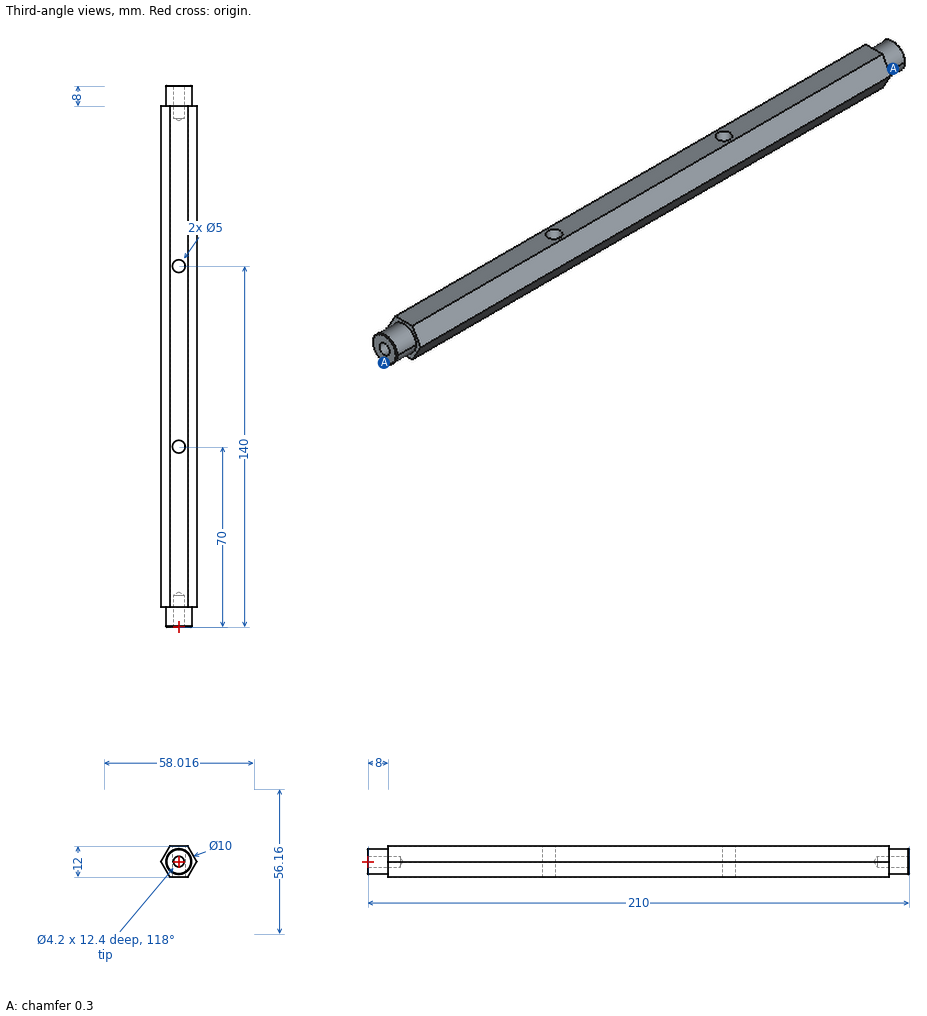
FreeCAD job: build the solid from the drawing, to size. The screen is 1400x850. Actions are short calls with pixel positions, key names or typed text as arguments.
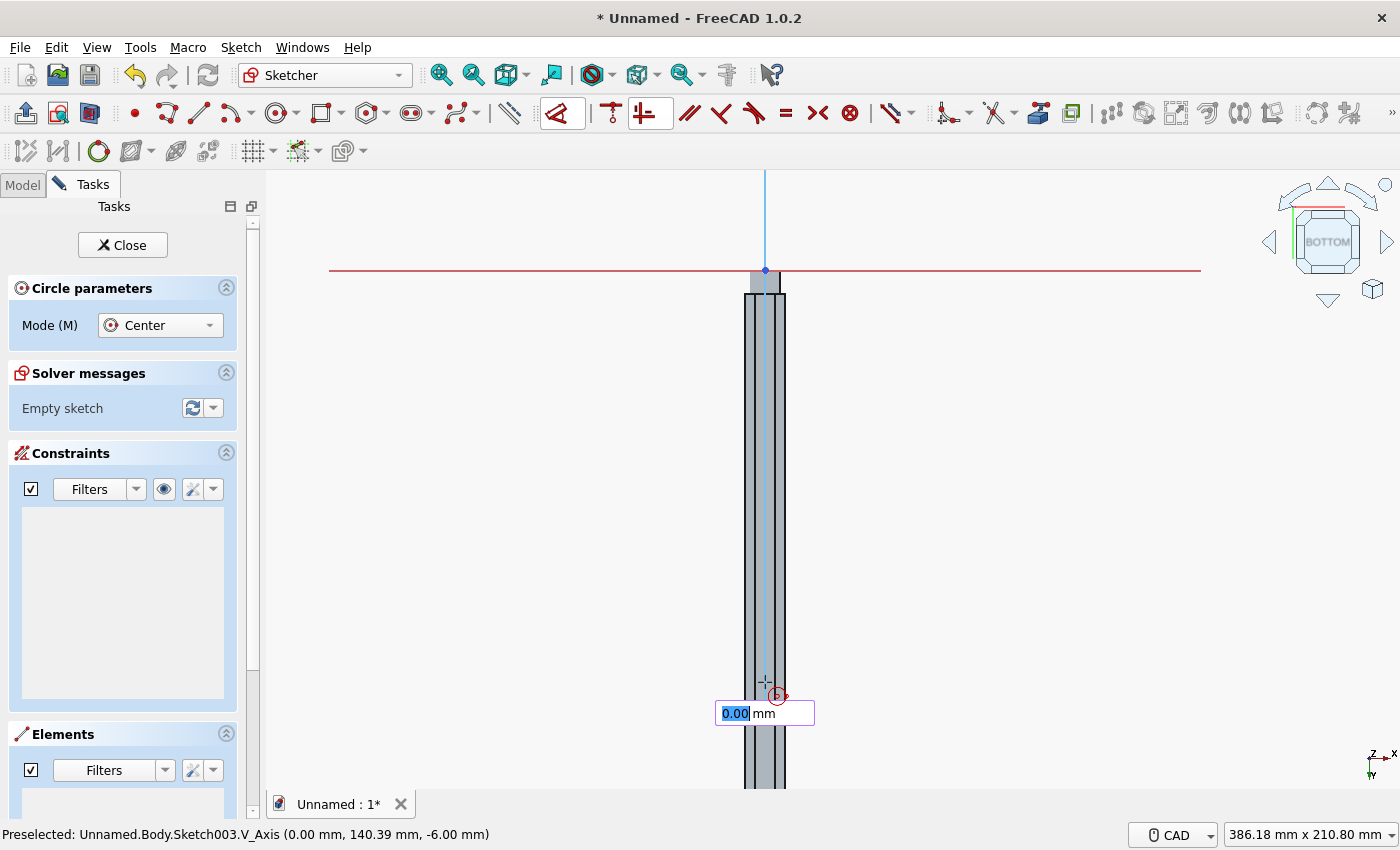
scroll(772, 679, up, 5)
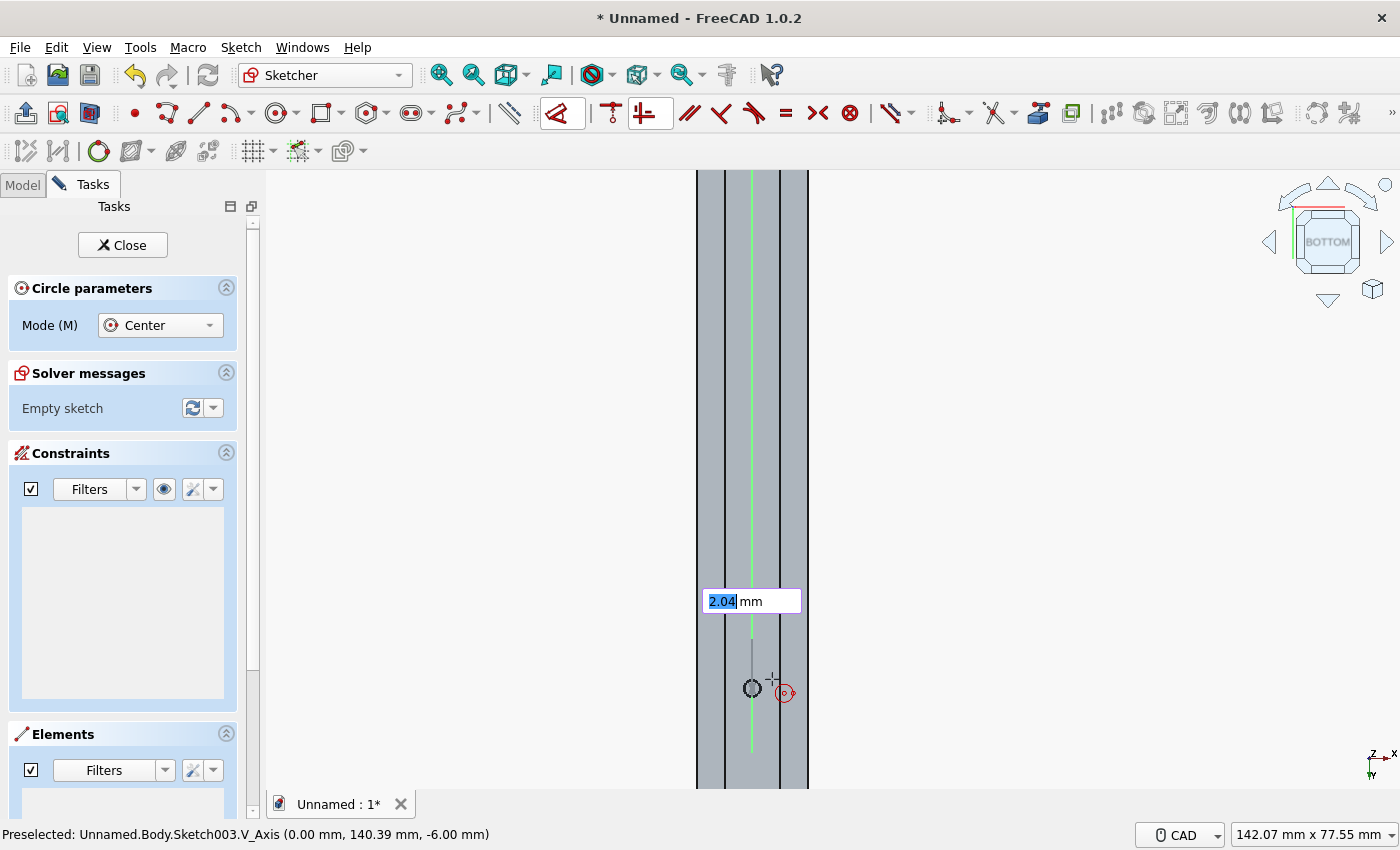
click(771, 678)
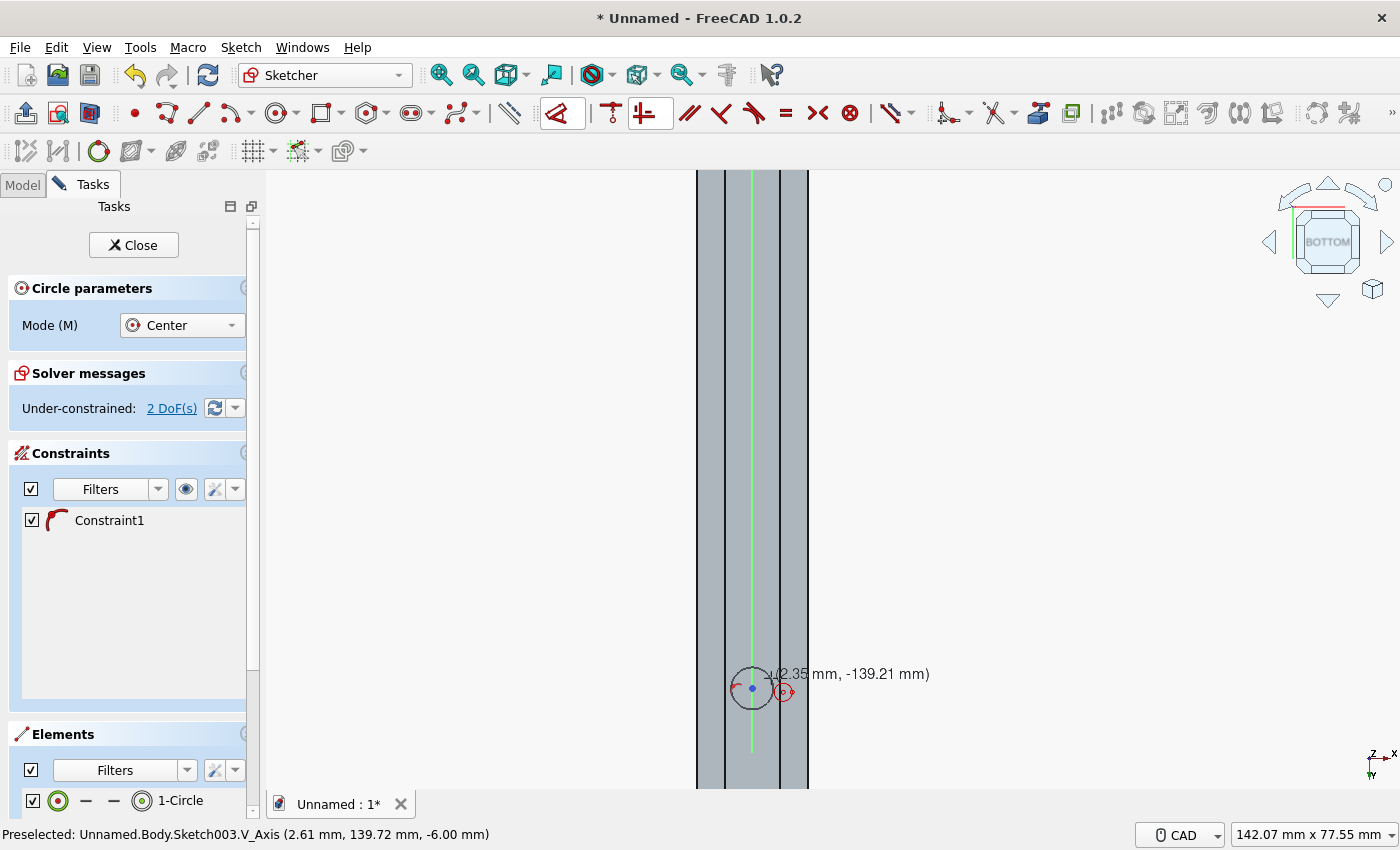
scroll(772, 679, down, 5)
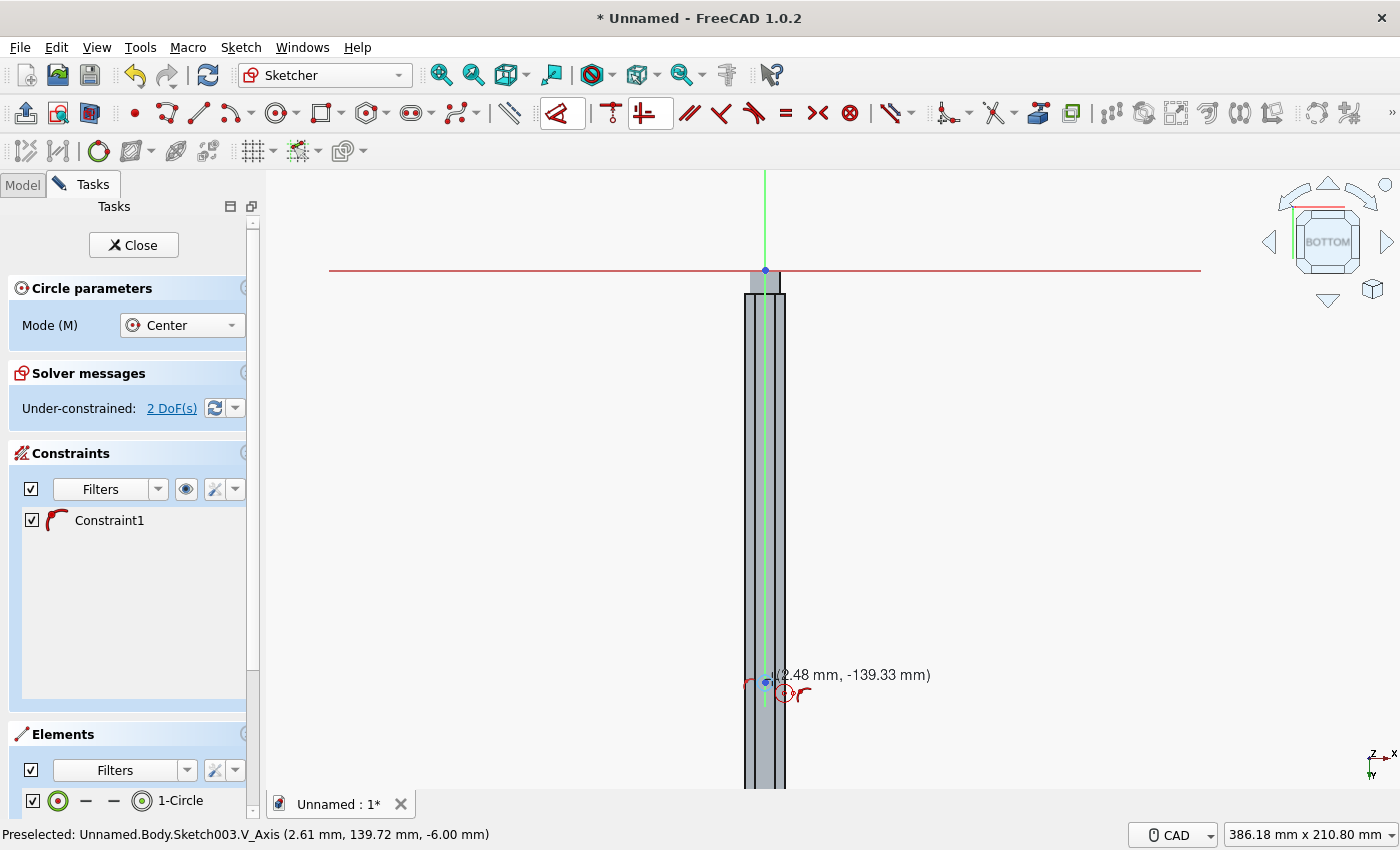
scroll(765, 476, up, 6)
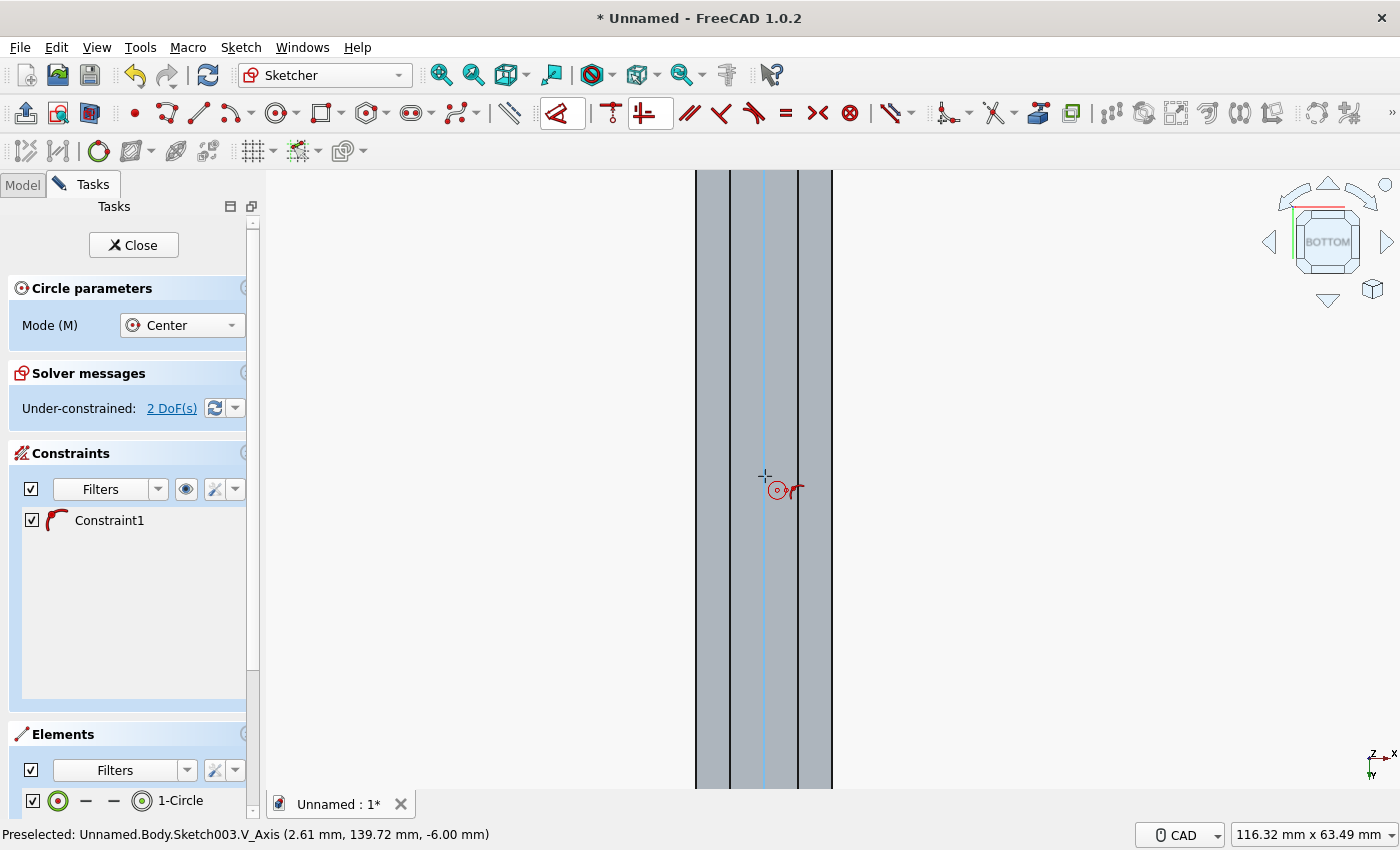
scroll(765, 476, down, 6)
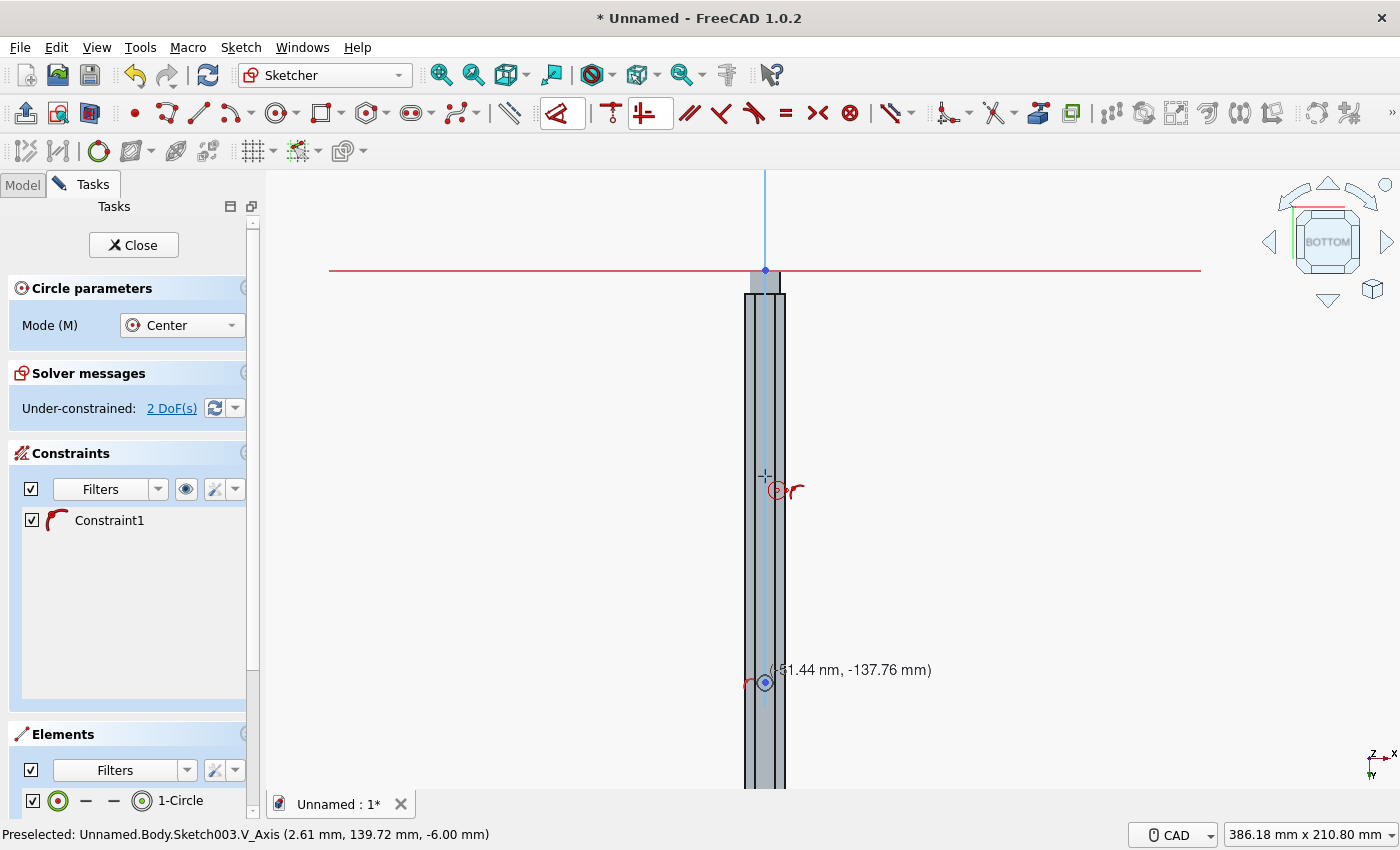
click(765, 476)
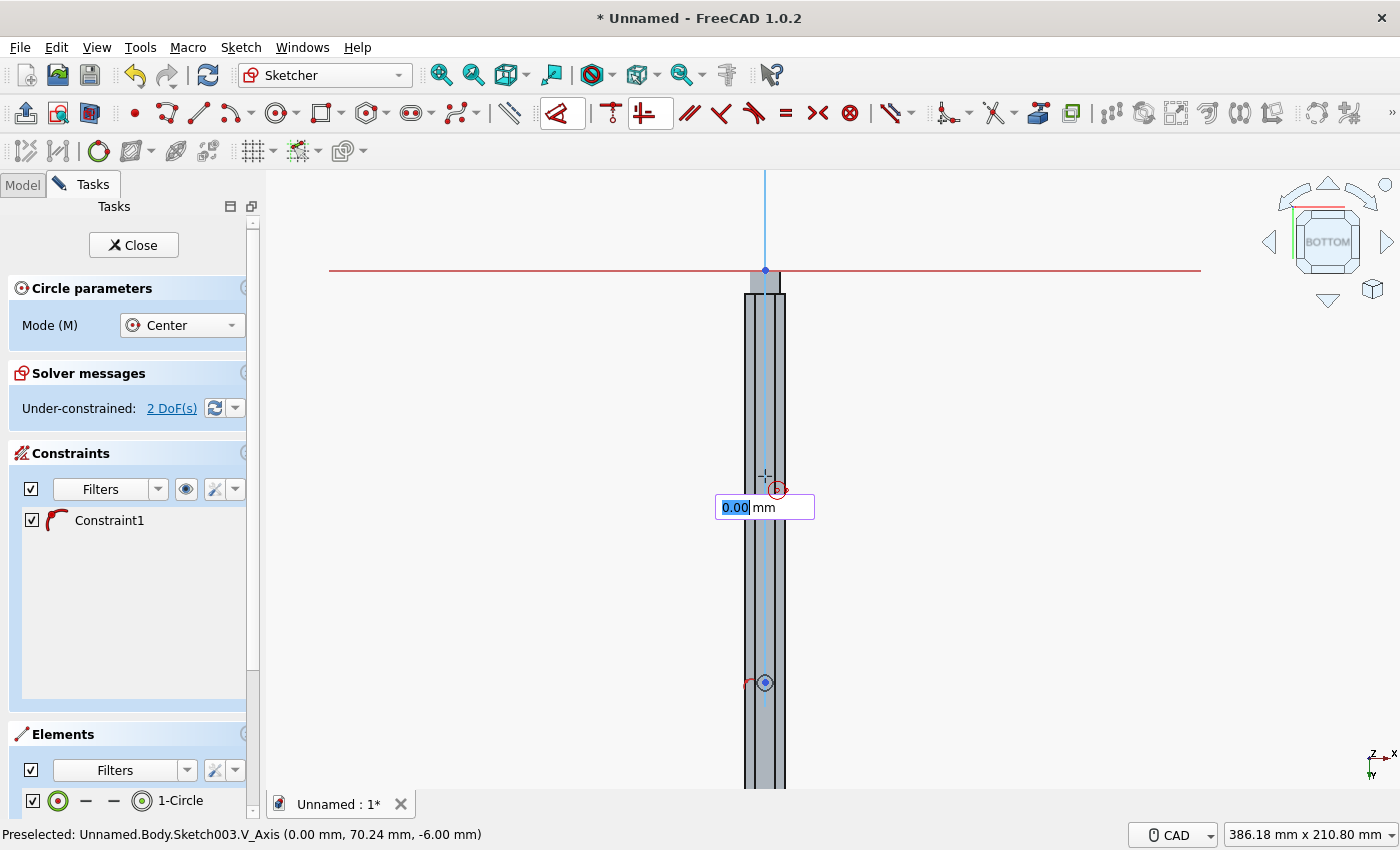
scroll(772, 474, up, 5)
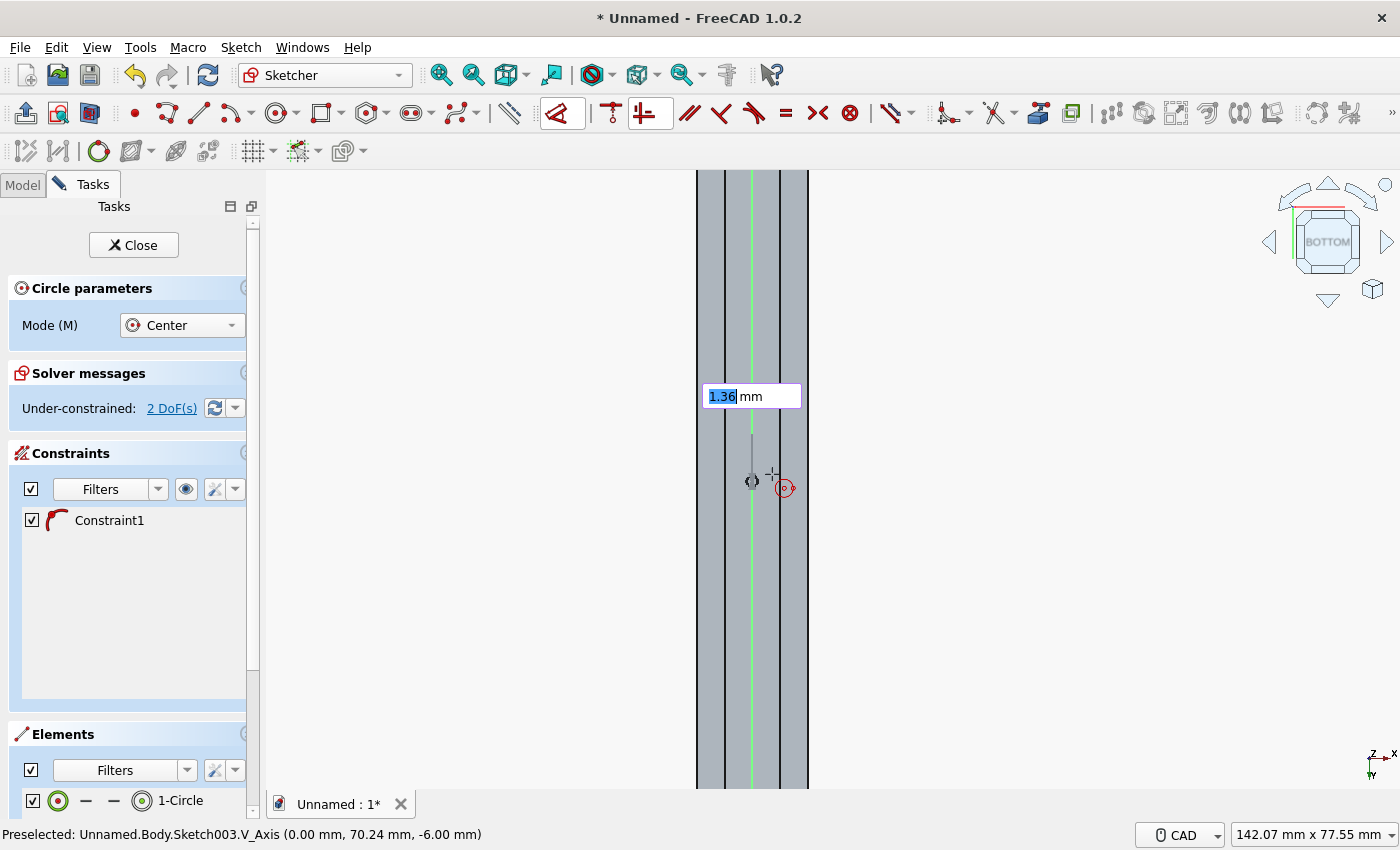
click(771, 473)
key(Escape)